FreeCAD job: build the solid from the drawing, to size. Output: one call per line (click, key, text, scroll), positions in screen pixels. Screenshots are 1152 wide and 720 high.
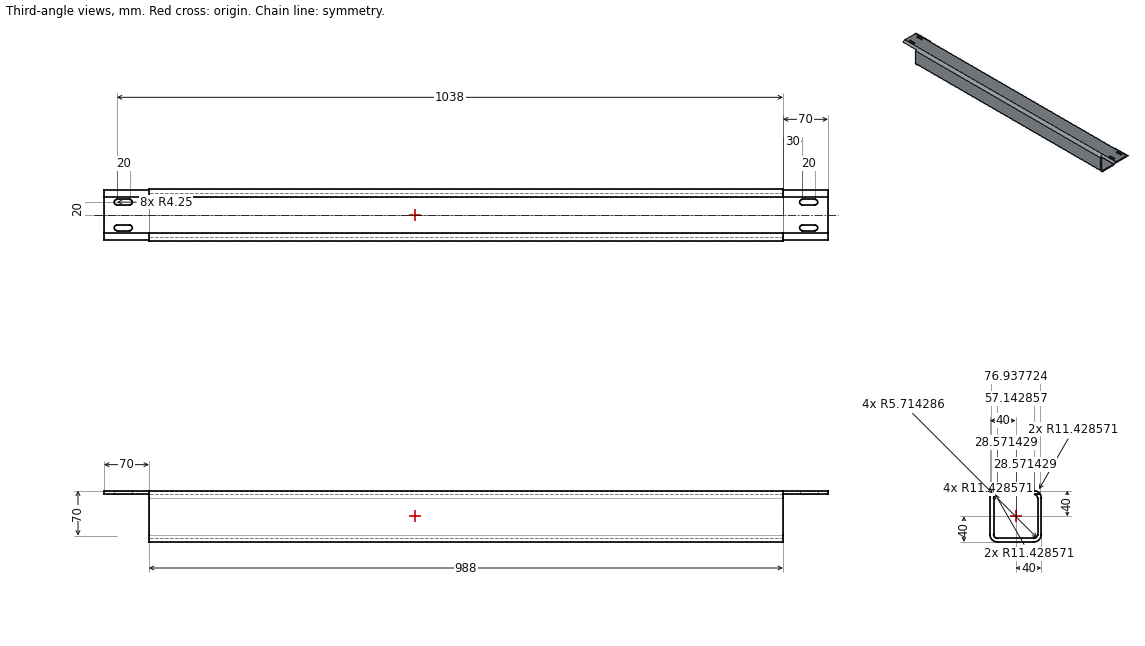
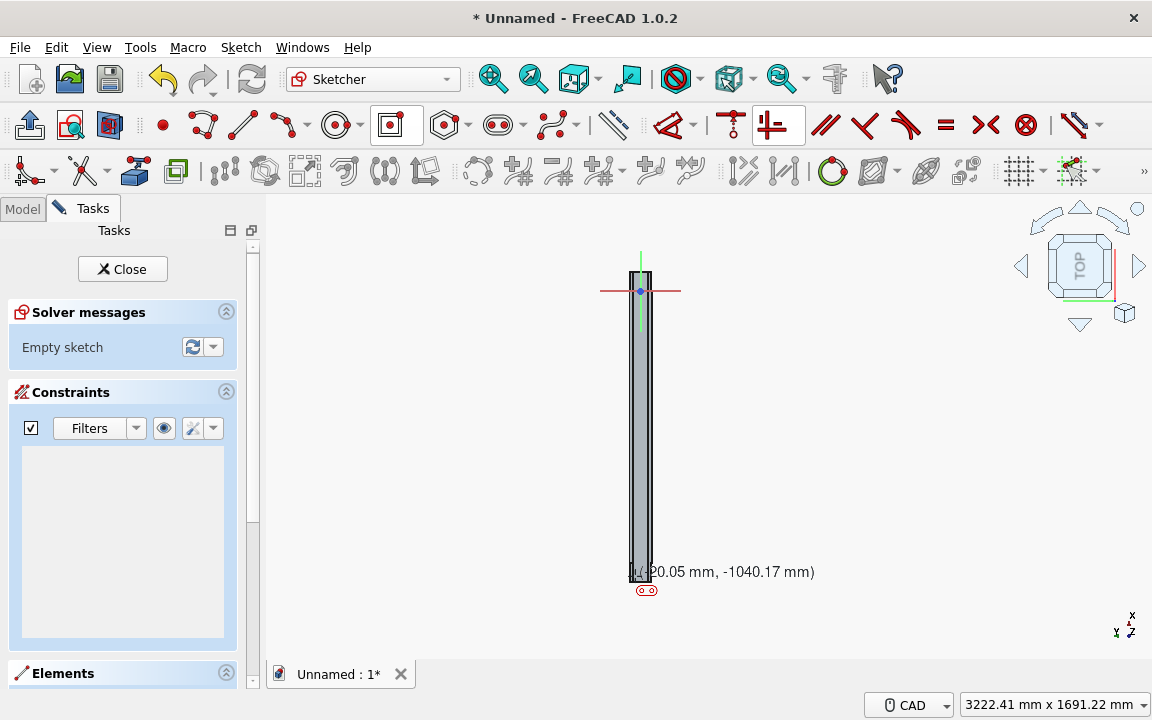
scroll(635, 576, up, 6)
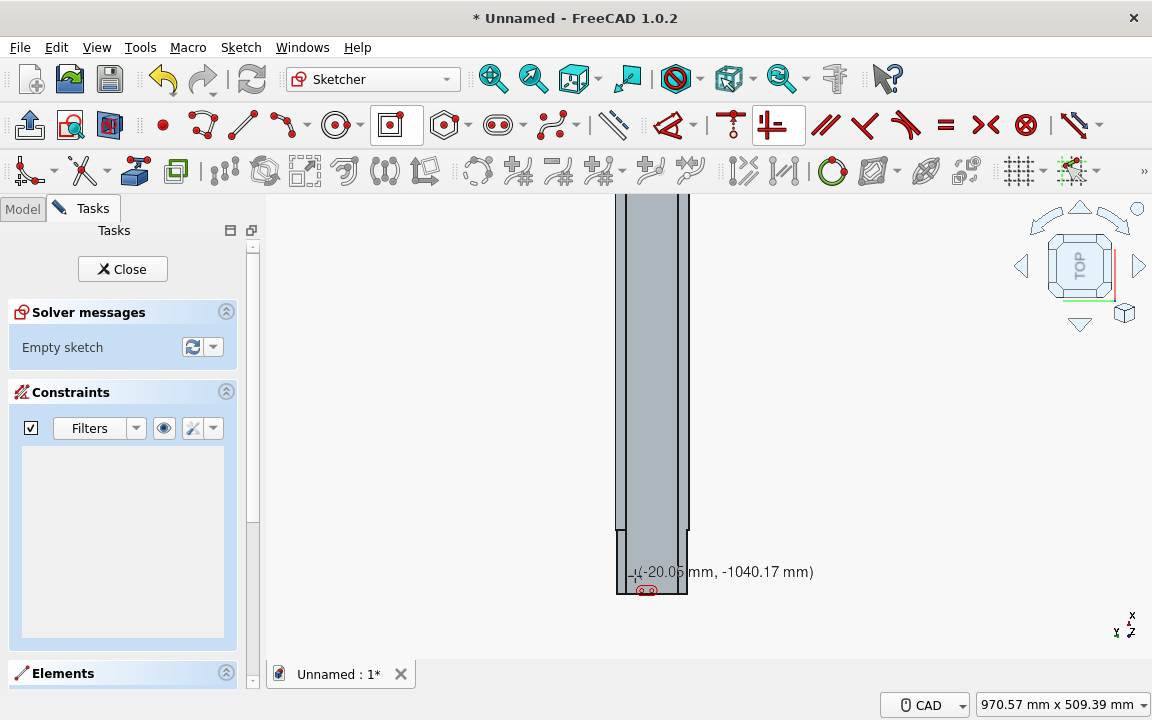
click(634, 575)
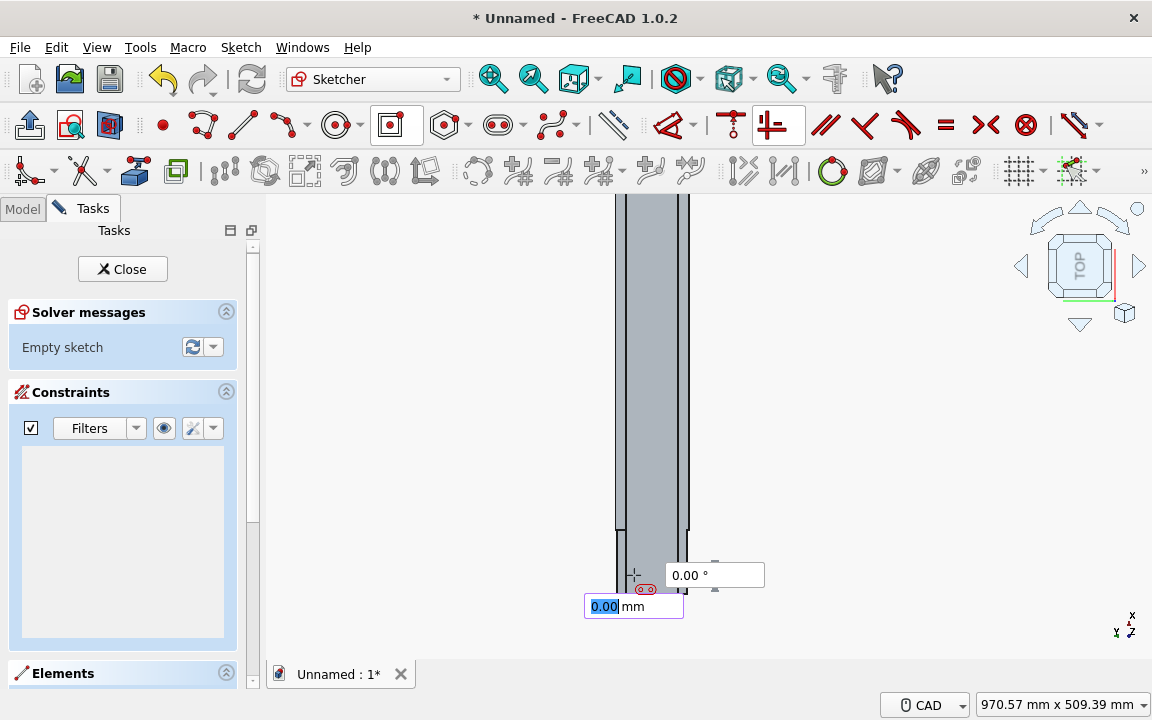
click(634, 557)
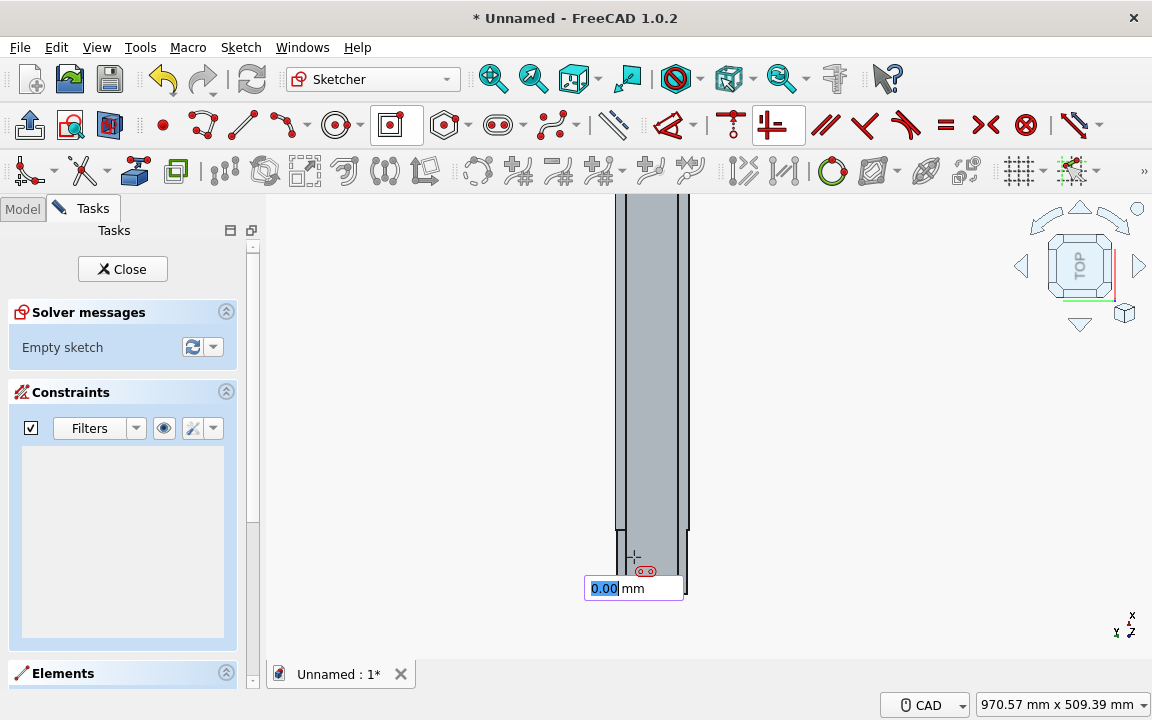
scroll(630, 566, up, 8)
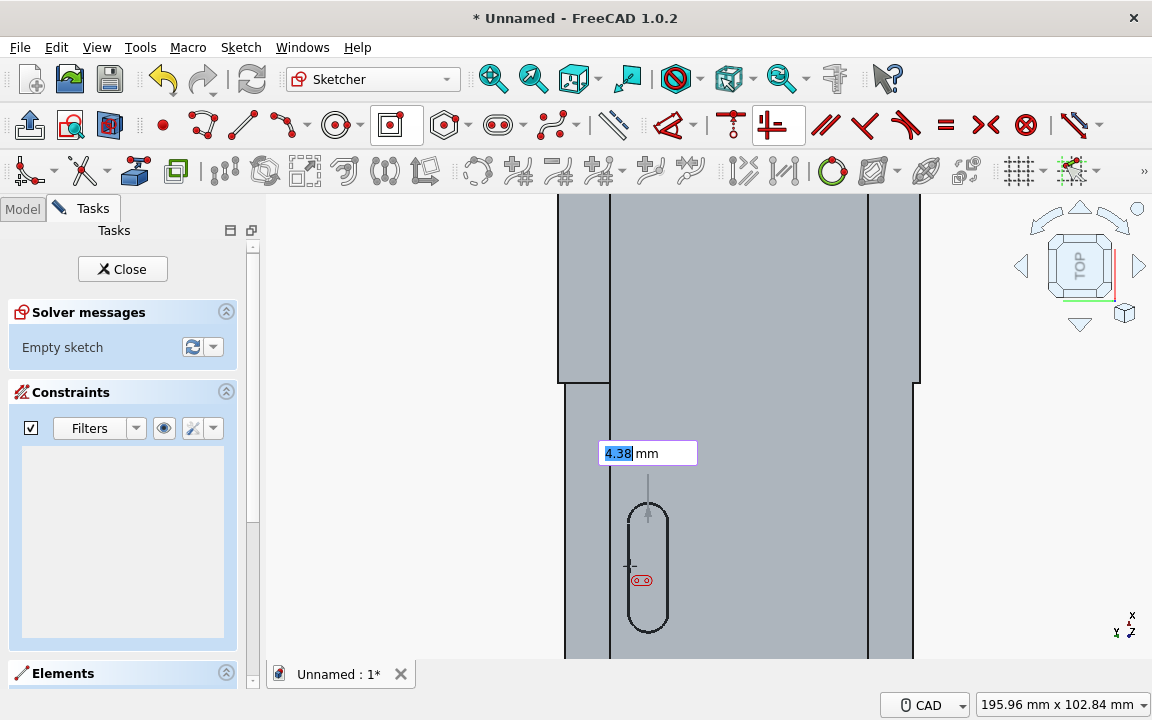
click(629, 564)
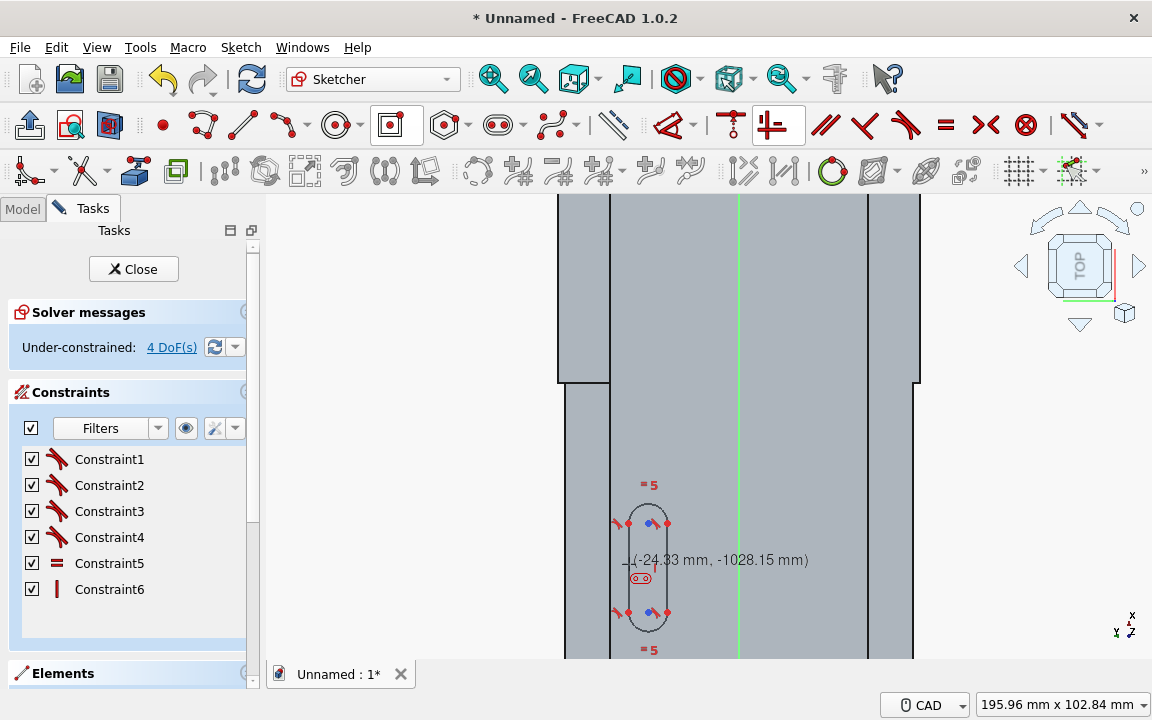
scroll(634, 574, down, 14)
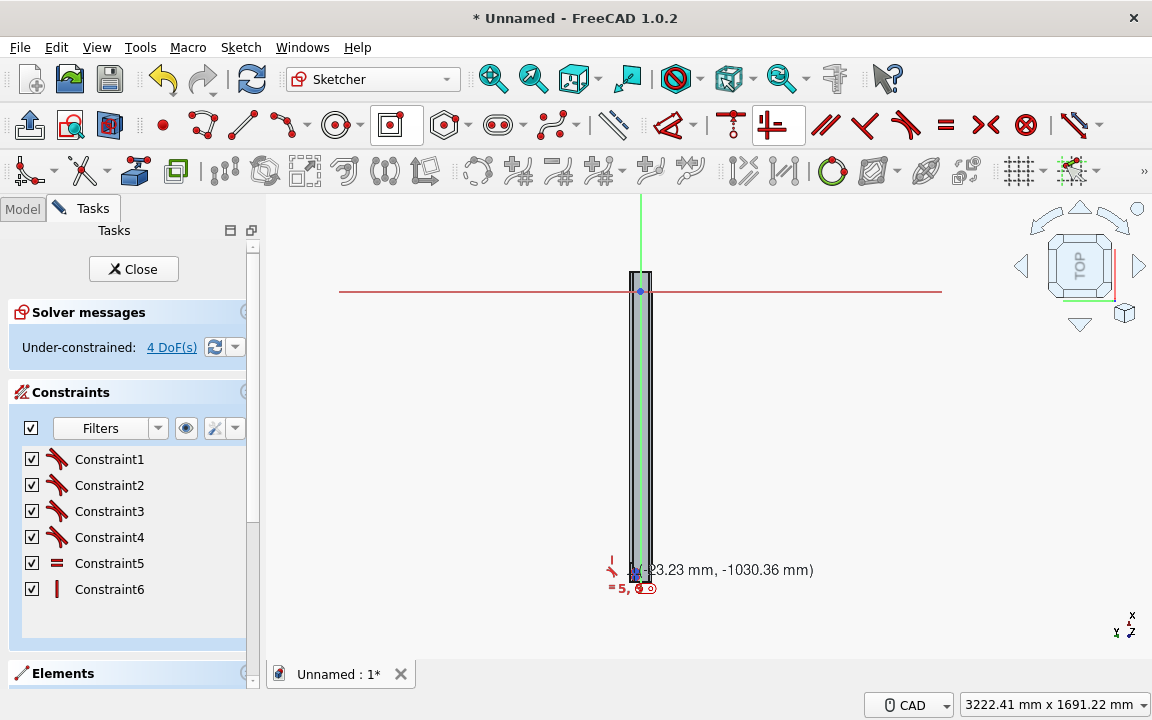
scroll(646, 577, up, 6)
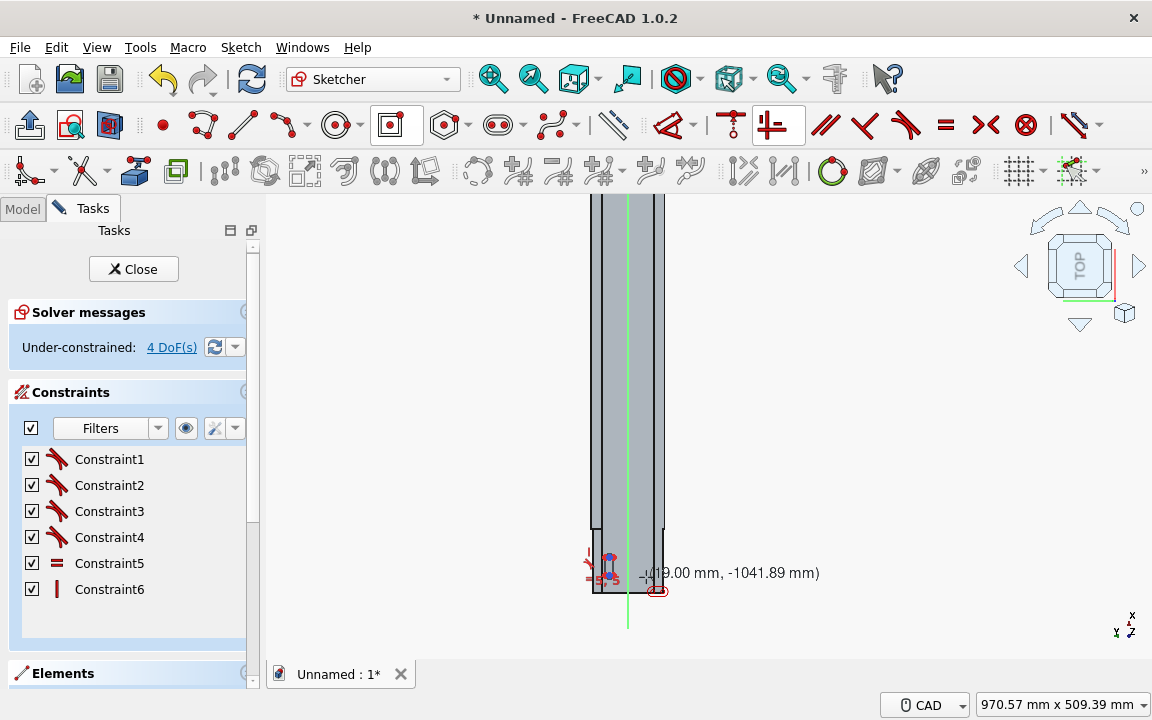
click(646, 575)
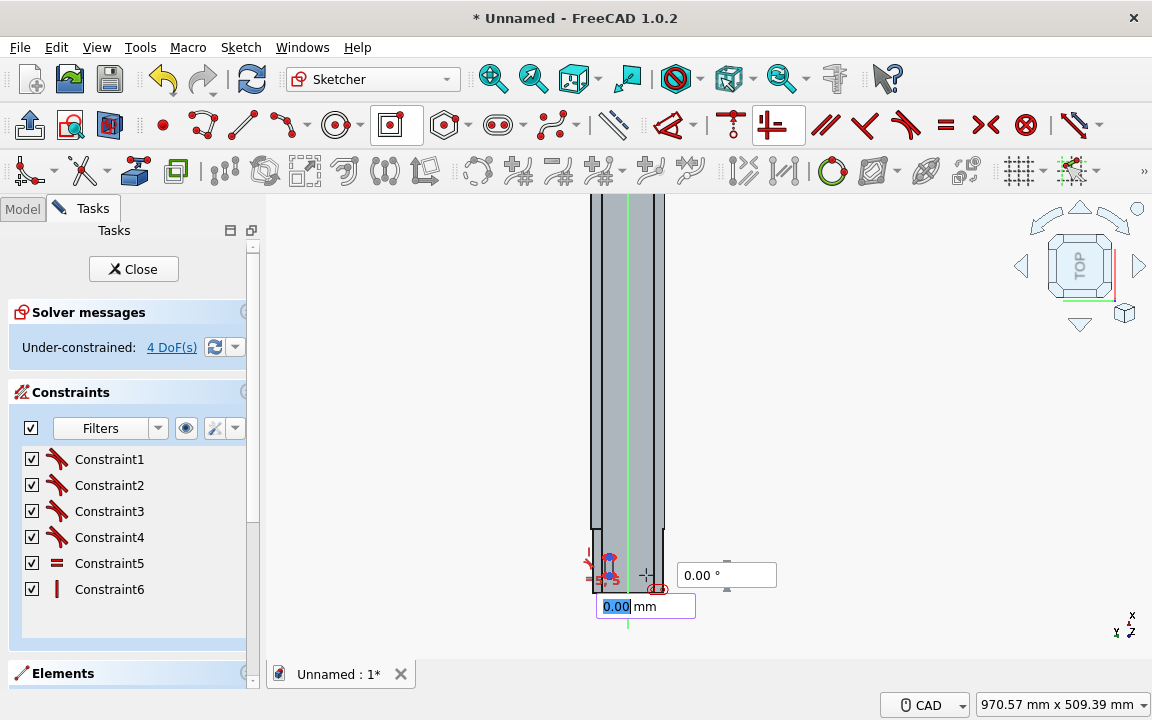
click(646, 557)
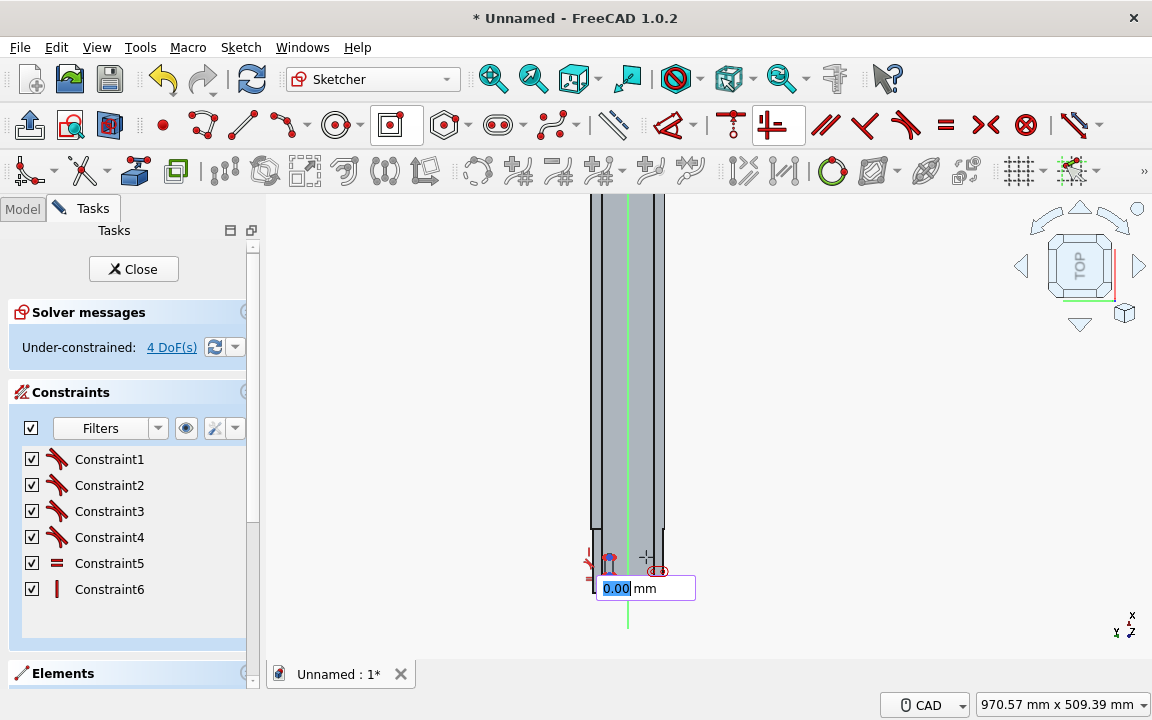
scroll(650, 566, up, 8)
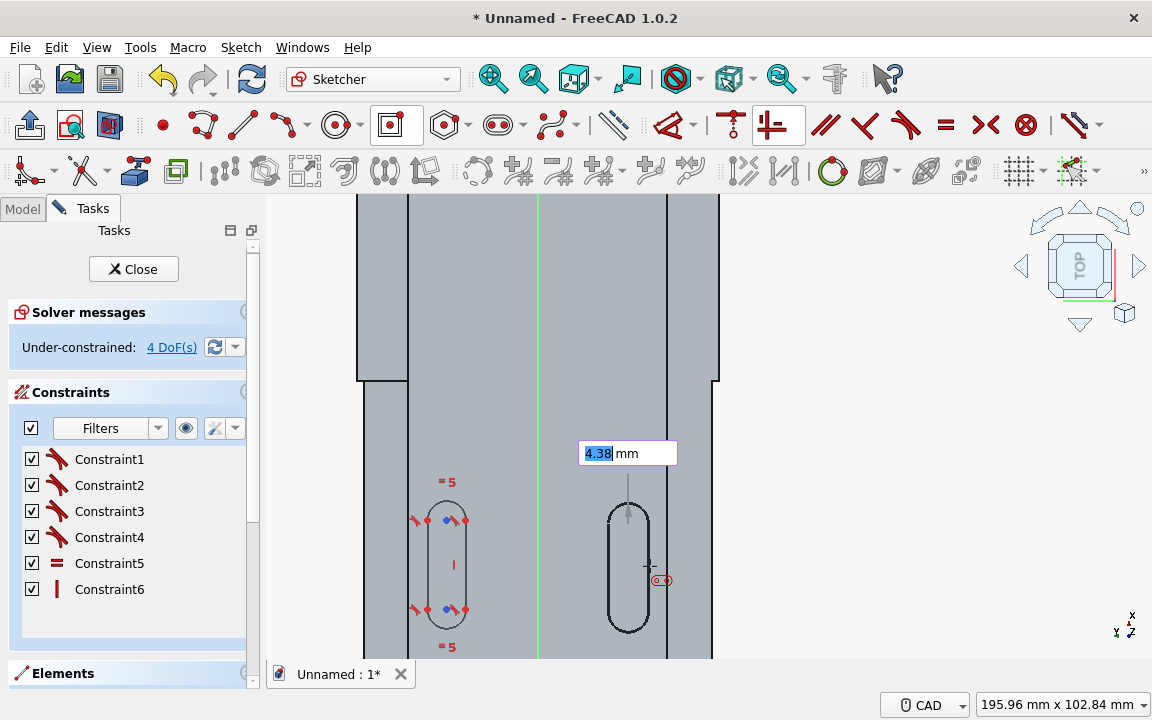
click(647, 561)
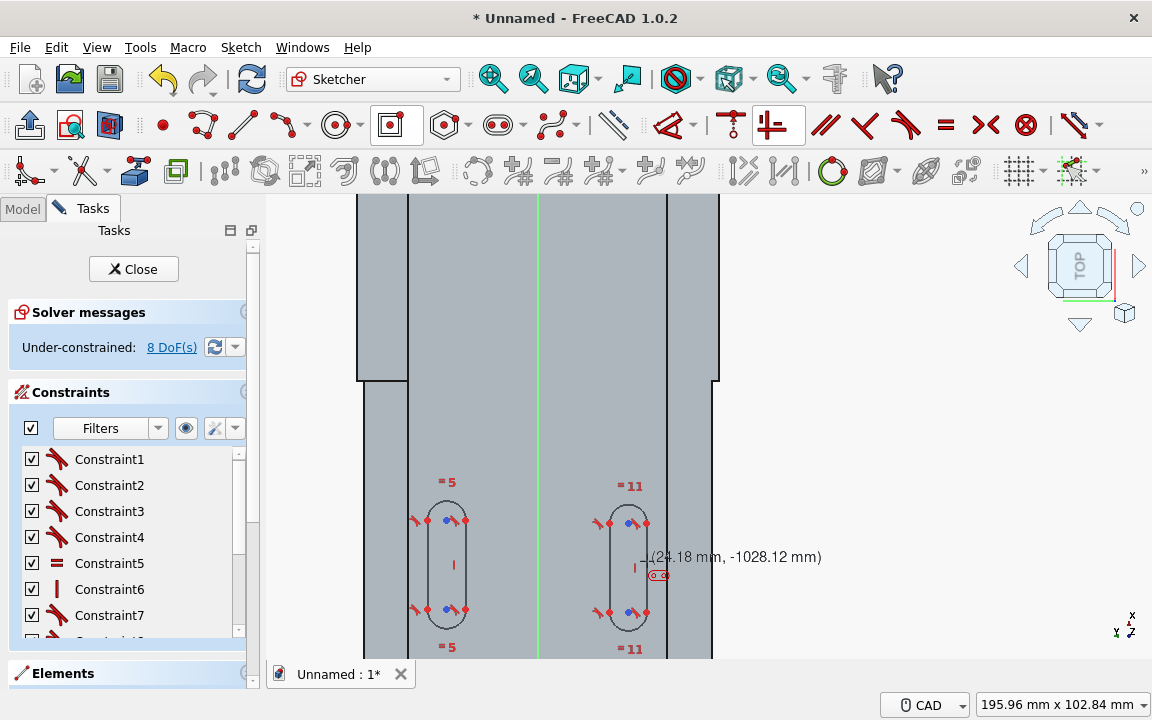
scroll(647, 574, down, 14)